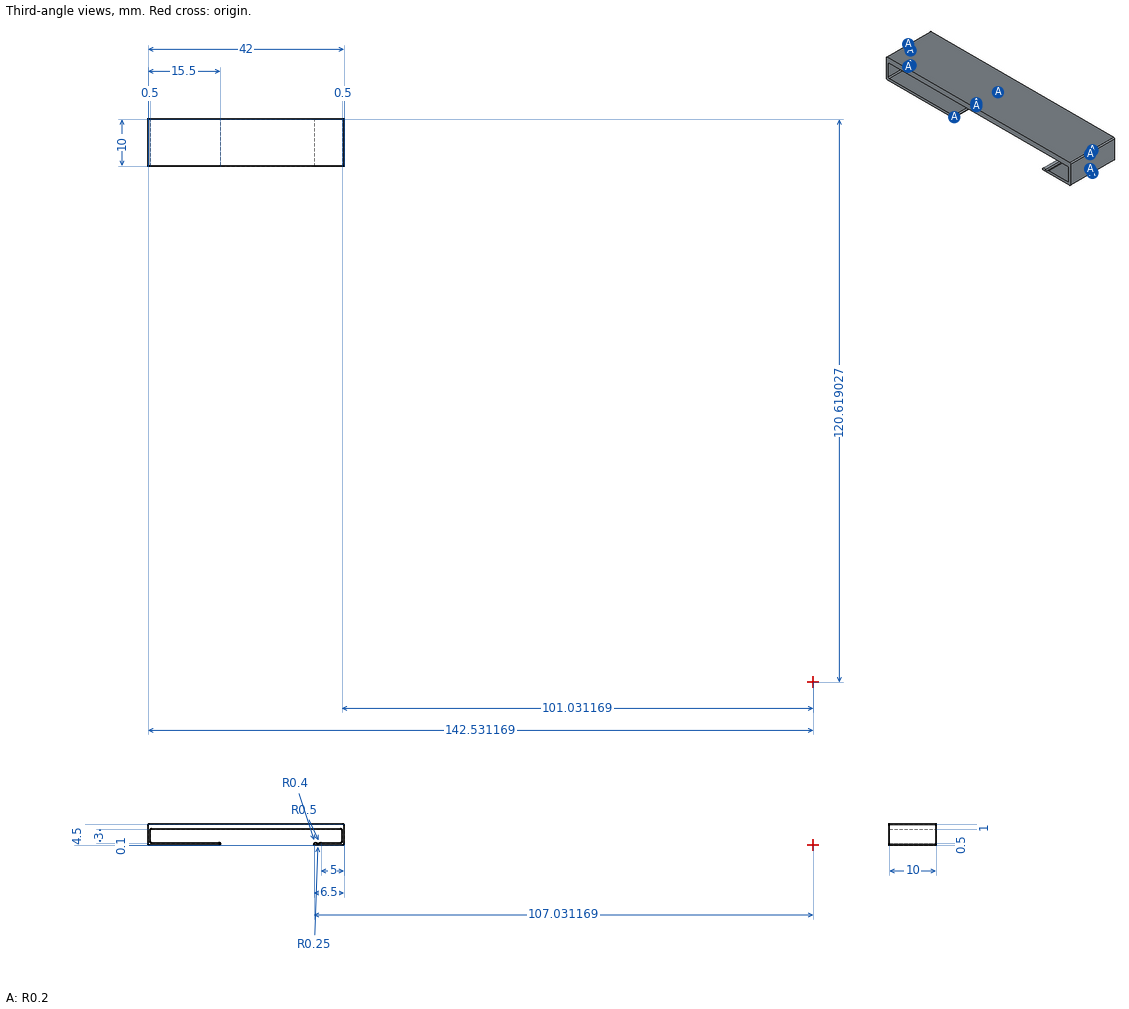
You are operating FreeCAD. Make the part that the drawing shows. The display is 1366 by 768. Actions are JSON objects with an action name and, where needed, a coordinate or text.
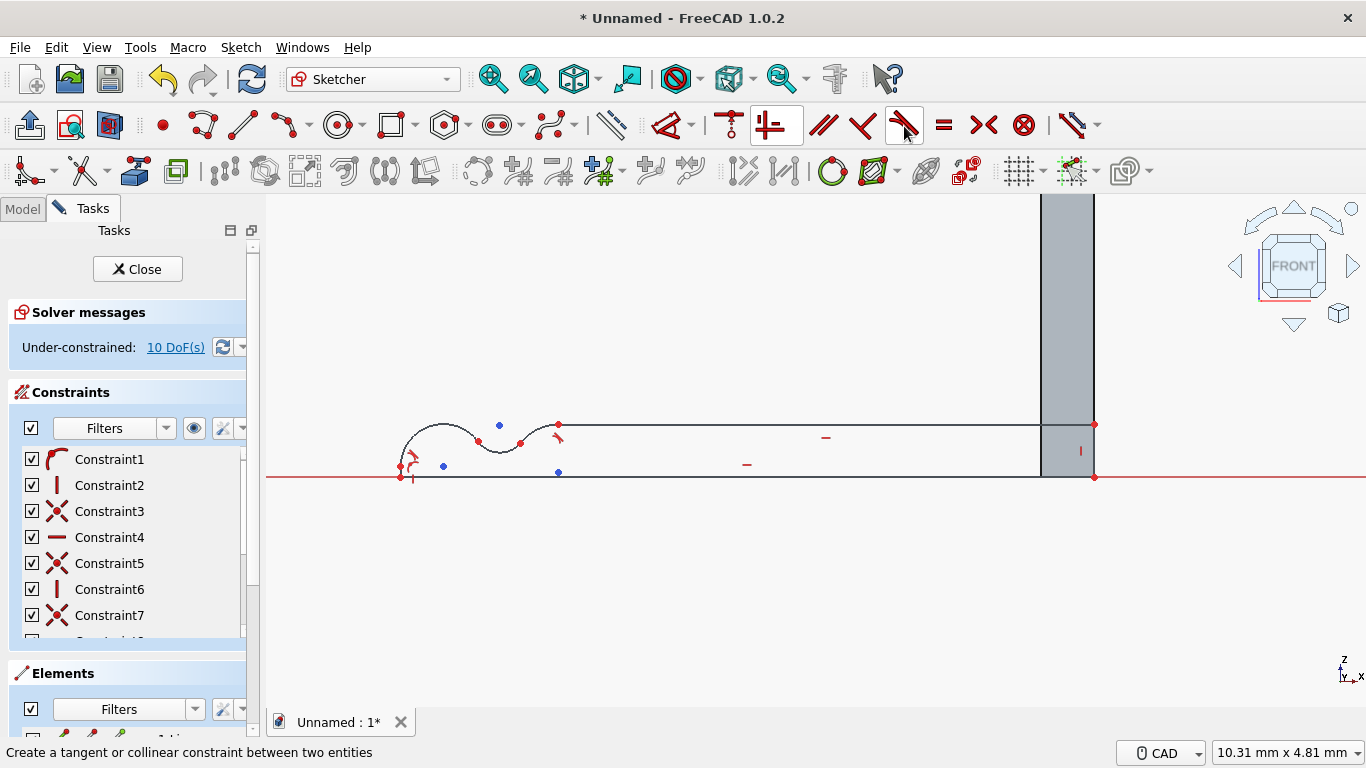
{"action": "left_click", "coordinate": [545, 426]}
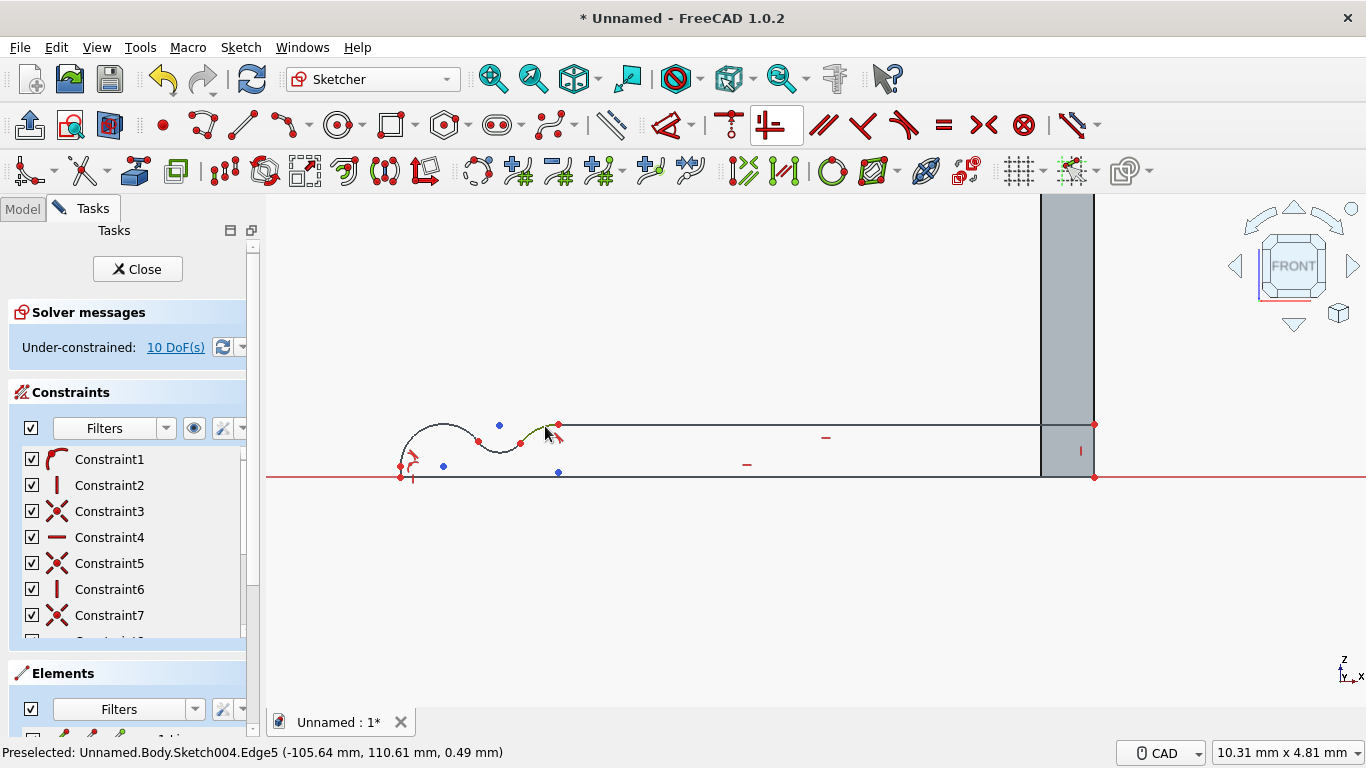
{"action": "left_click", "coordinate": [489, 450]}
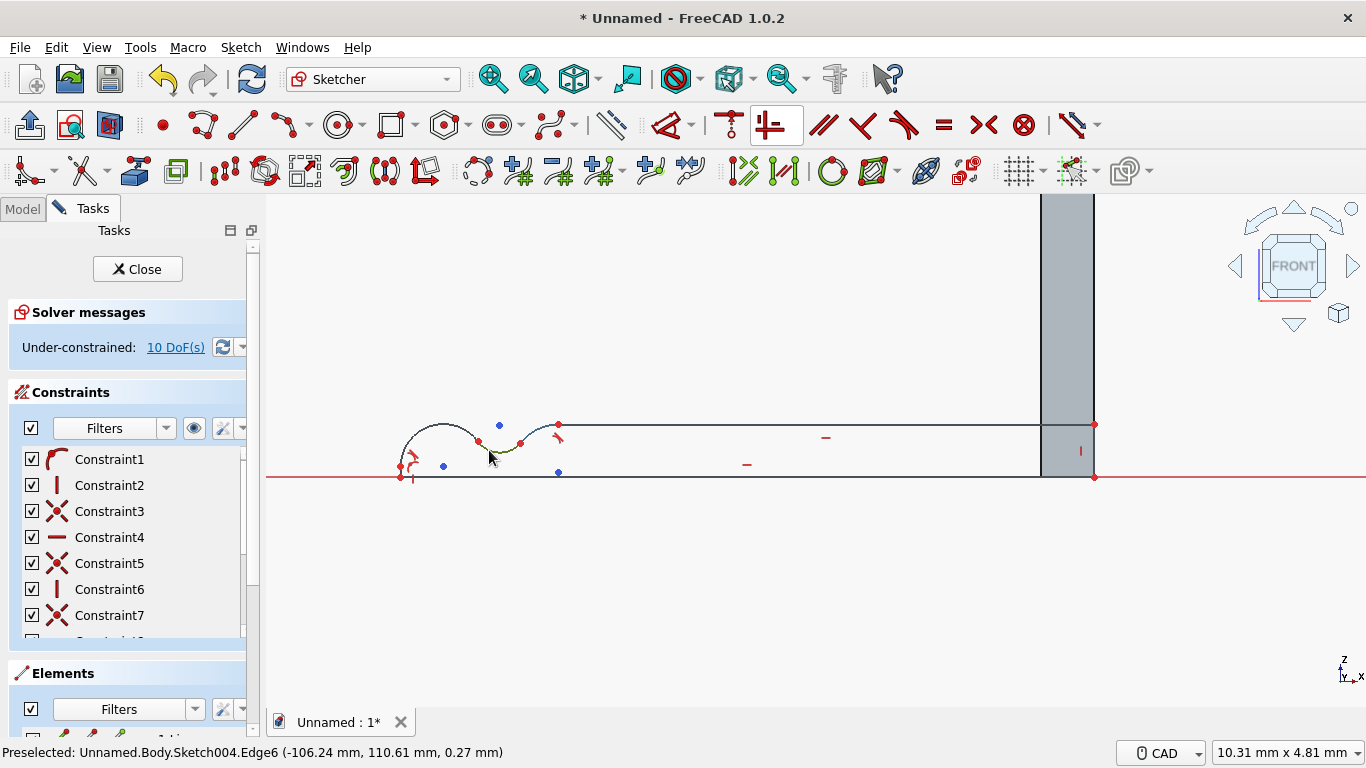
{"action": "left_click", "coordinate": [904, 126]}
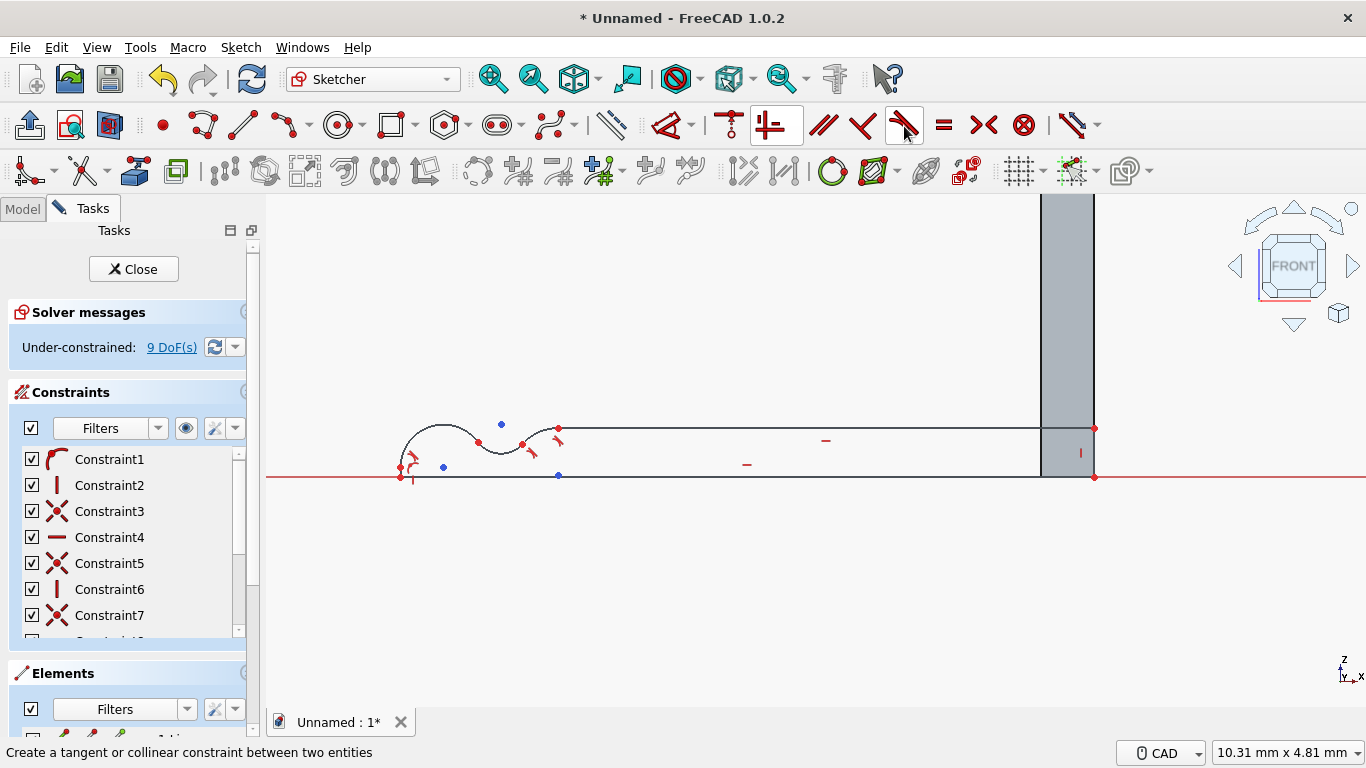
{"action": "left_click", "coordinate": [490, 451]}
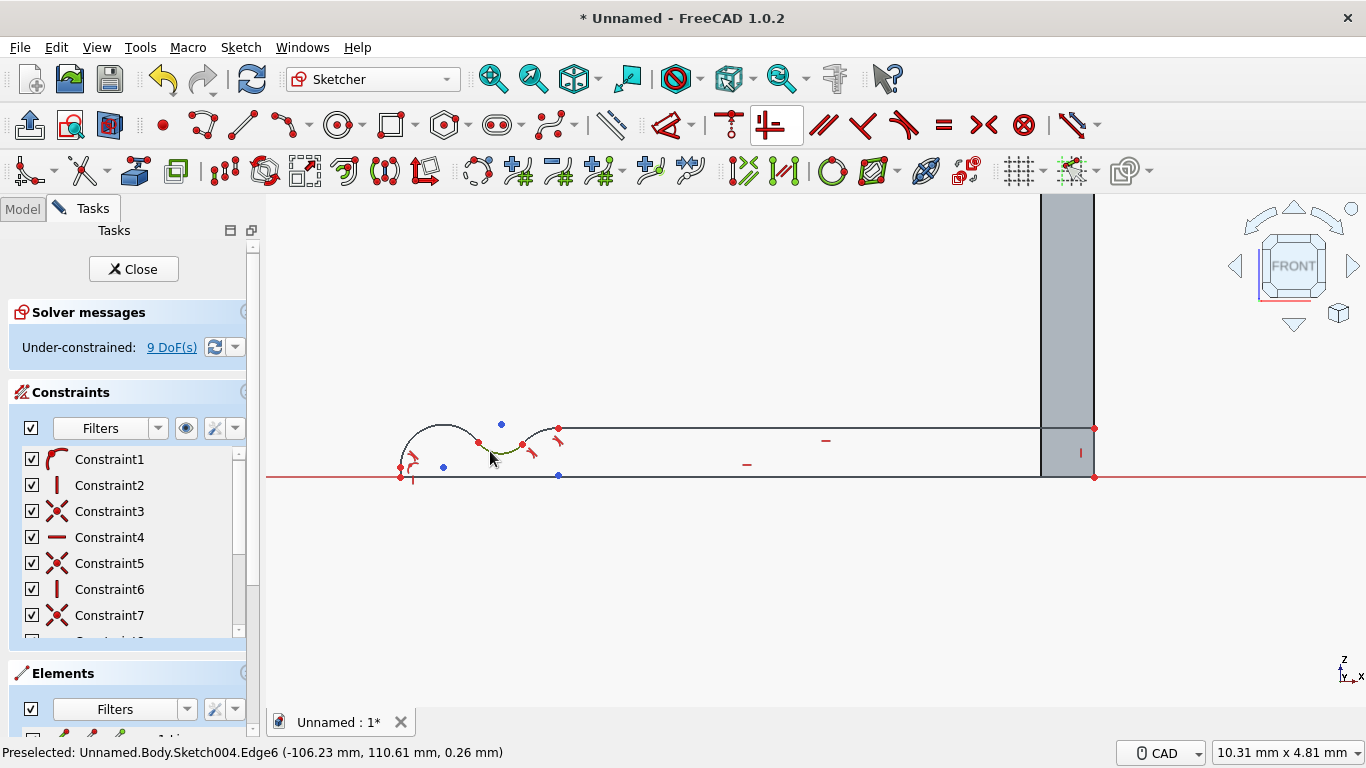
{"action": "left_click", "coordinate": [451, 425]}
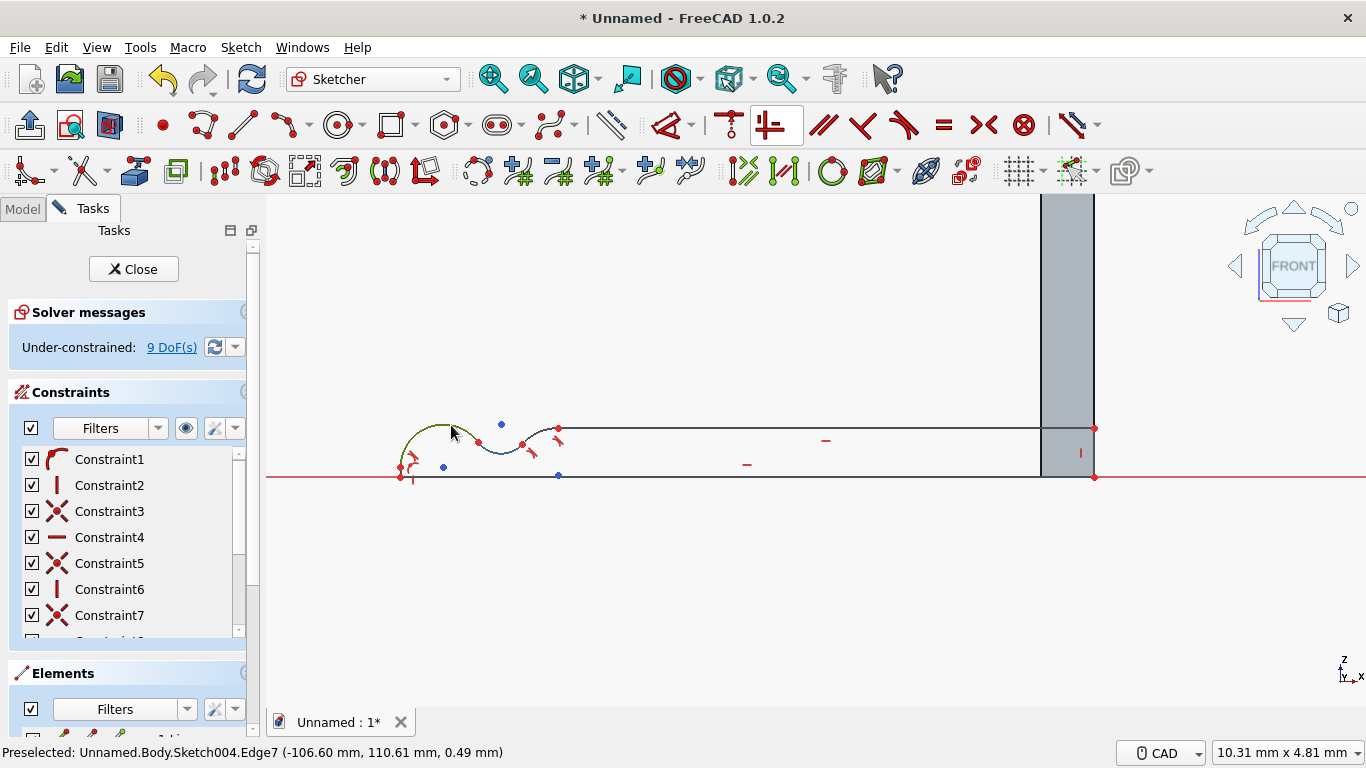
{"action": "left_click", "coordinate": [904, 126]}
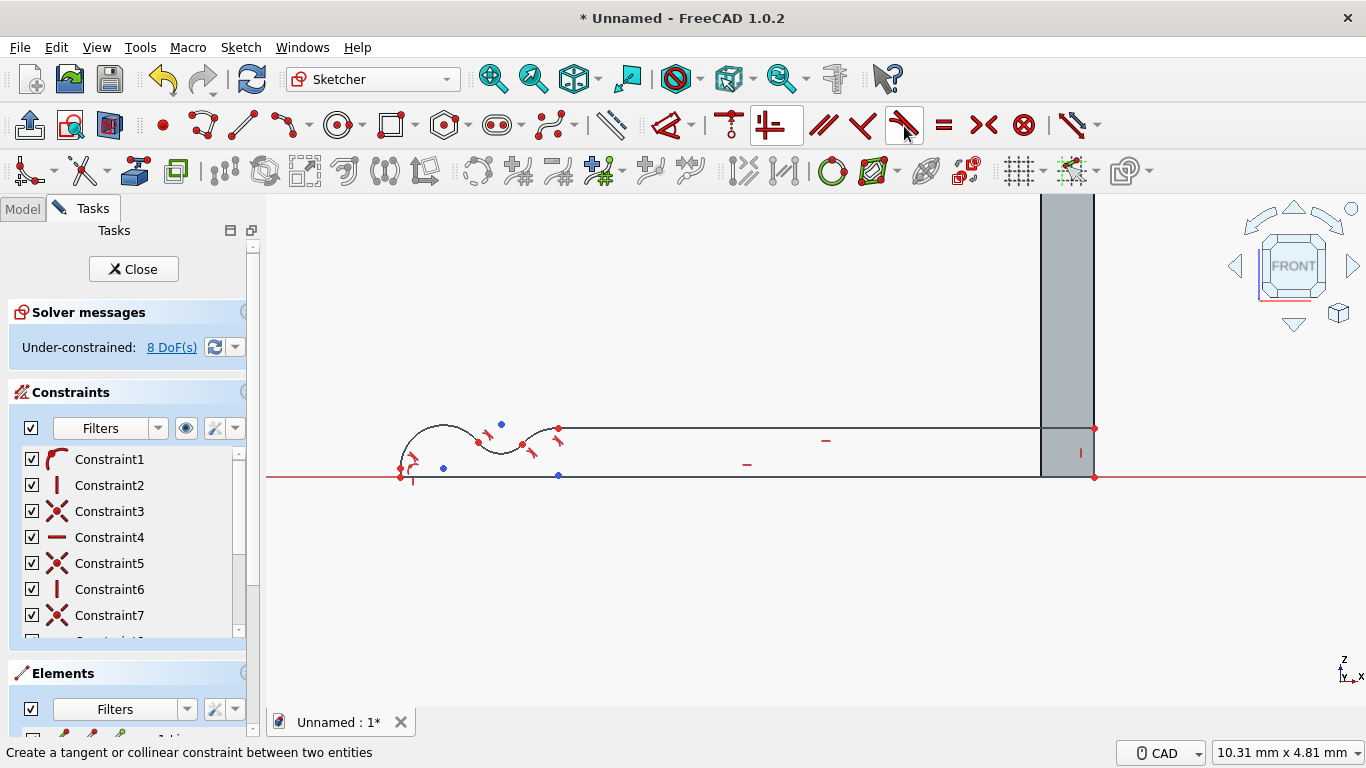
{"action": "left_click", "coordinate": [558, 476]}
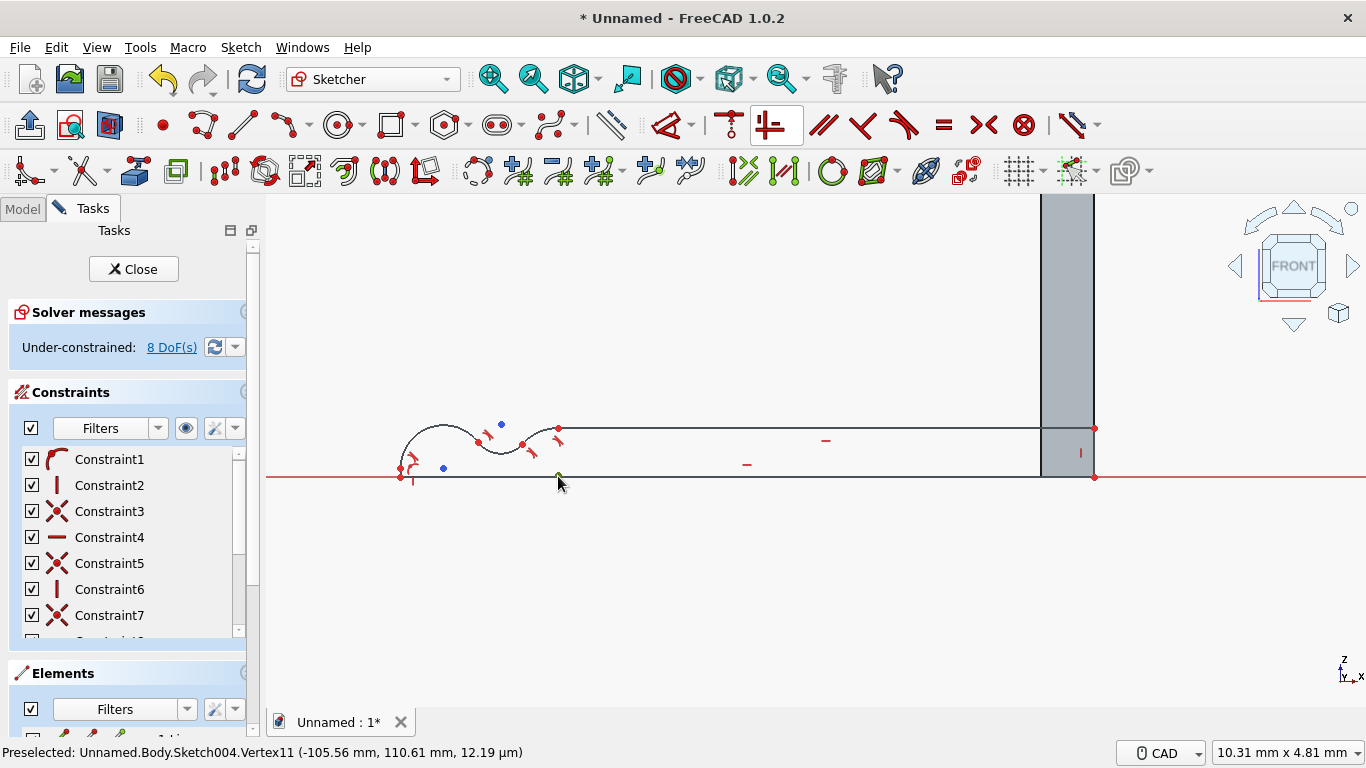
{"action": "left_click", "coordinate": [359, 477]}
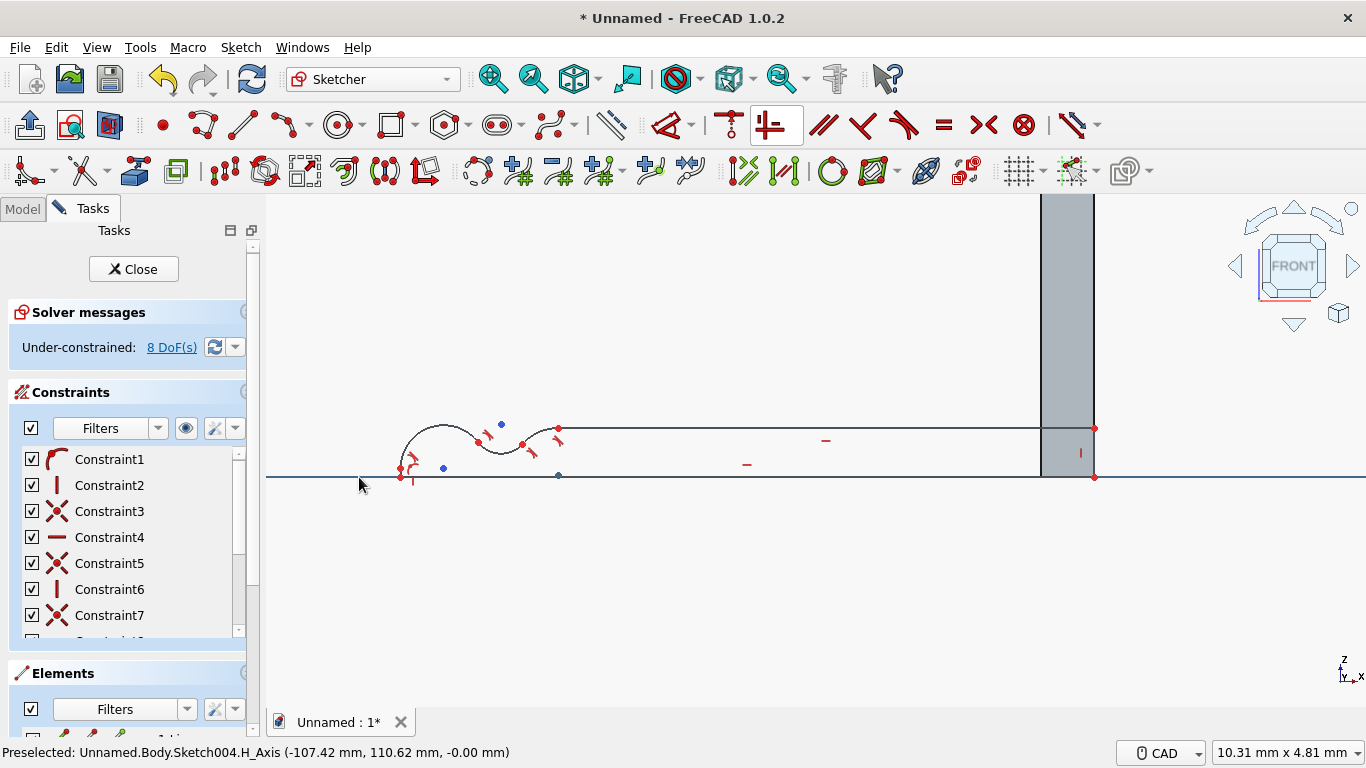
{"action": "left_click", "coordinate": [730, 126]}